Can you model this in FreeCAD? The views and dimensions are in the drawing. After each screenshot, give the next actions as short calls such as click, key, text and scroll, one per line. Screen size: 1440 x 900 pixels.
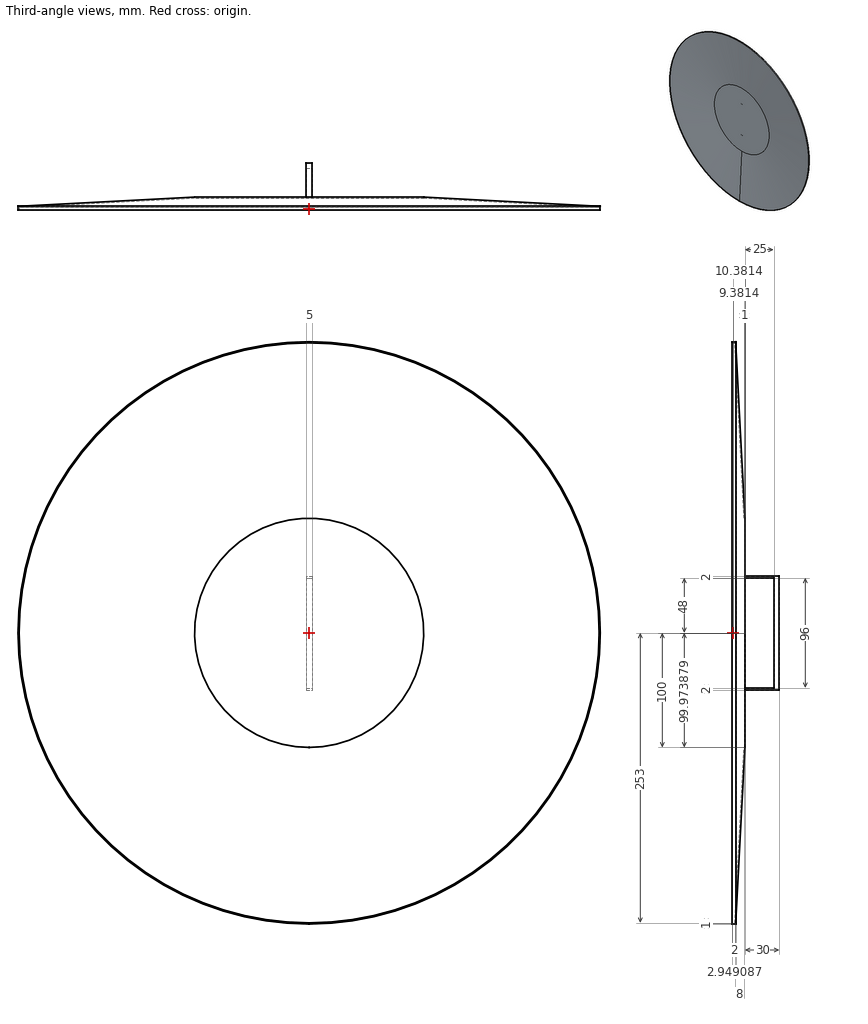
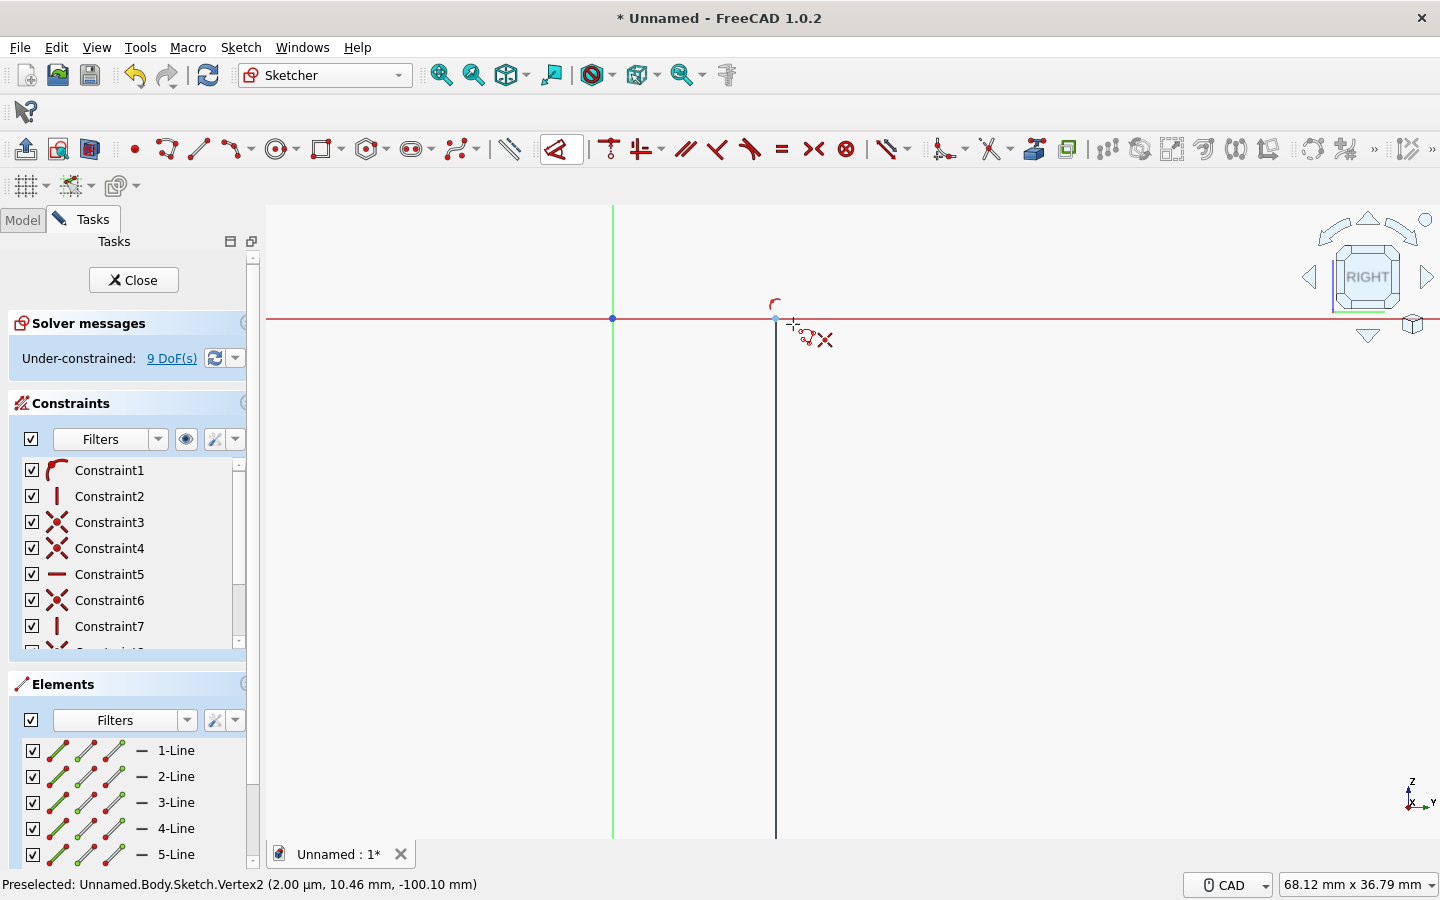
click(792, 328)
click(776, 319)
key(Escape)
key(Escape)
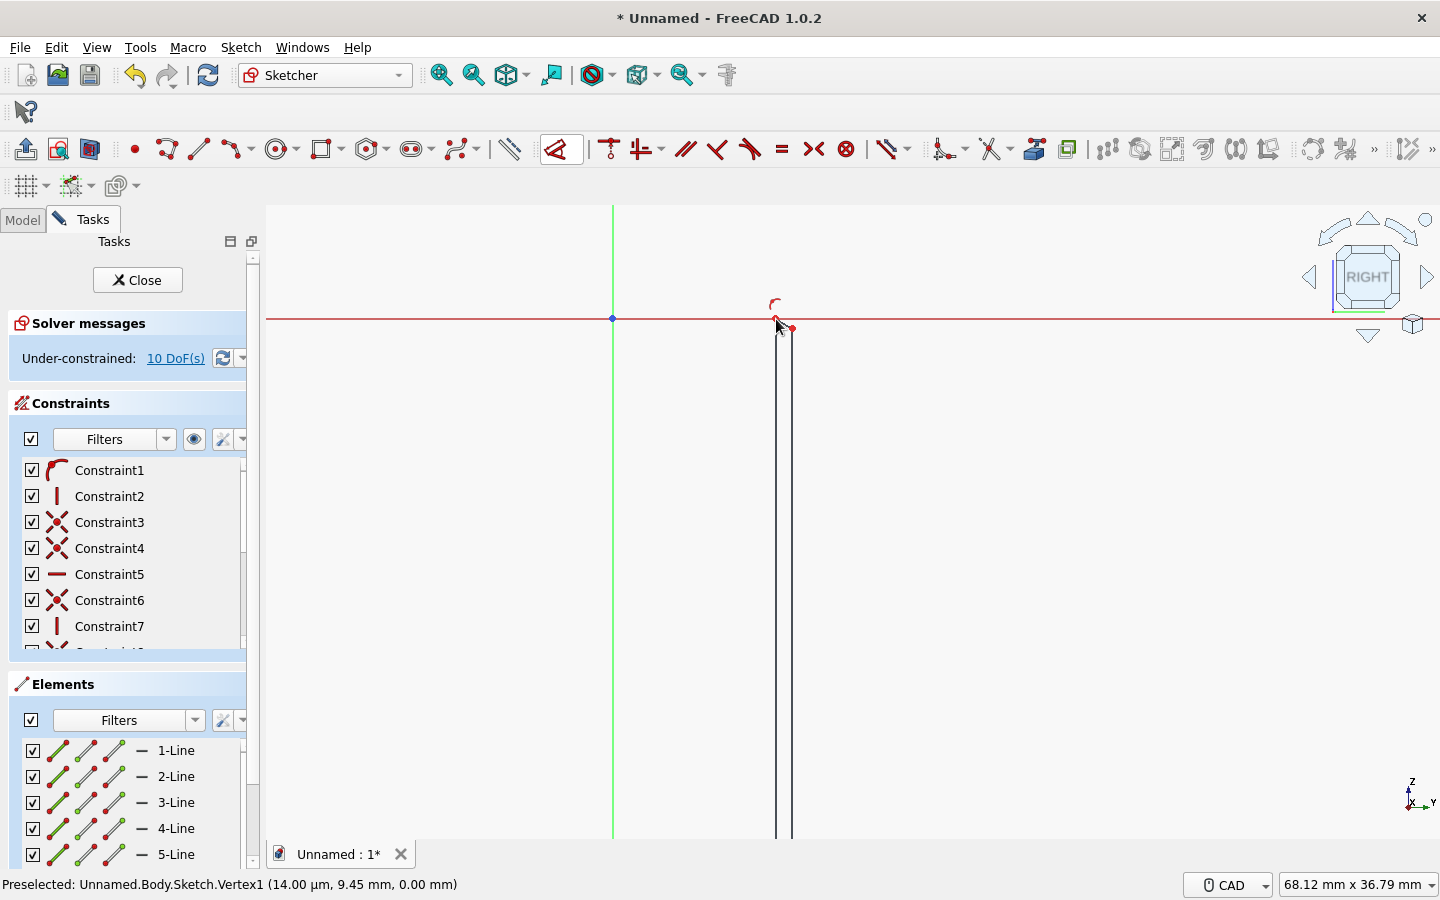
scroll(782, 323, up, 2)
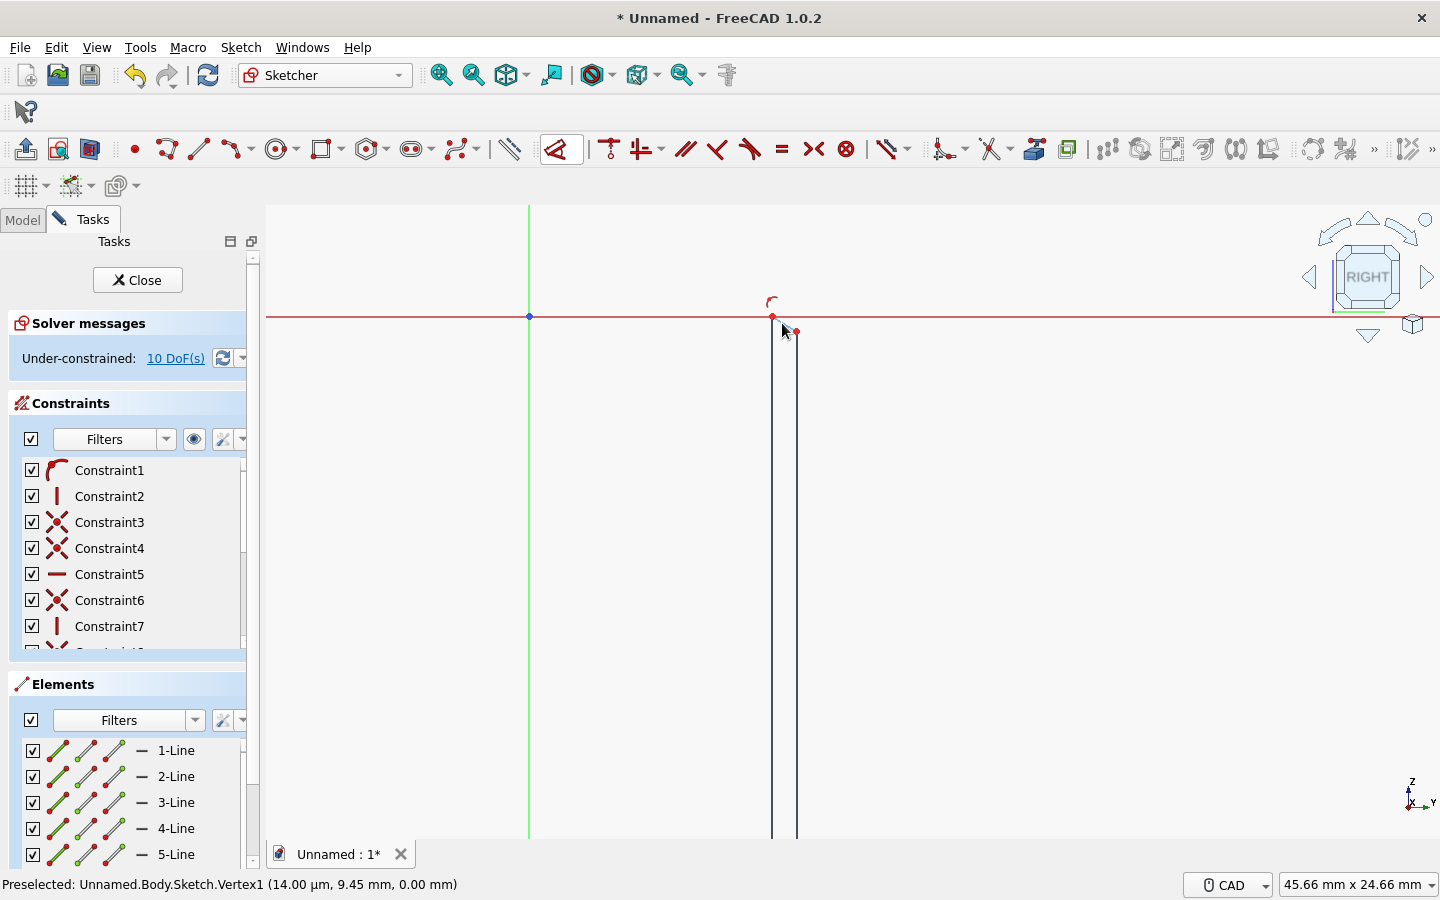
click(782, 323)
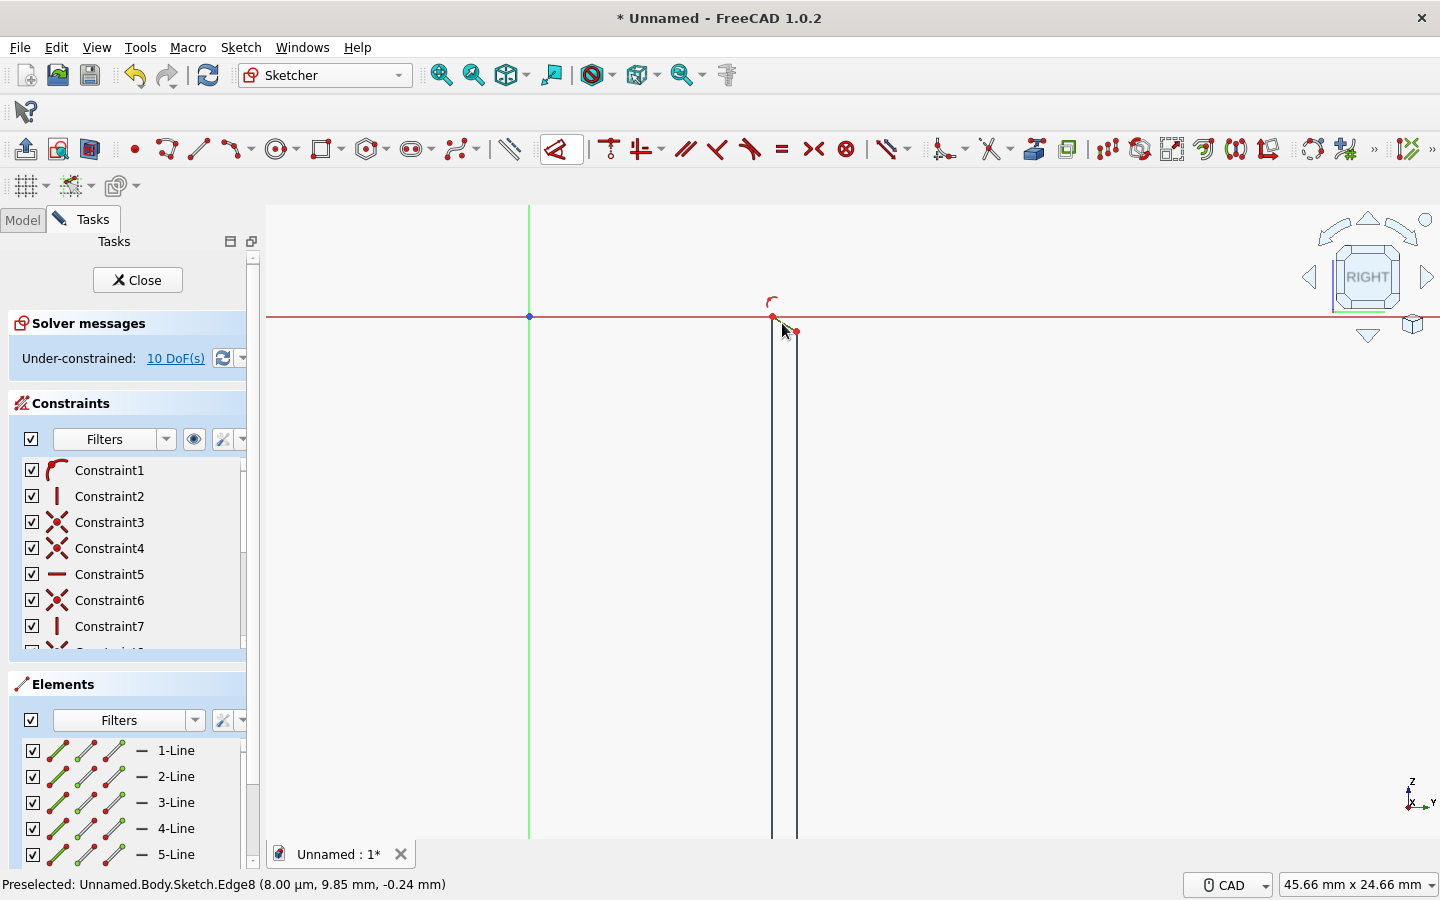
click(664, 150)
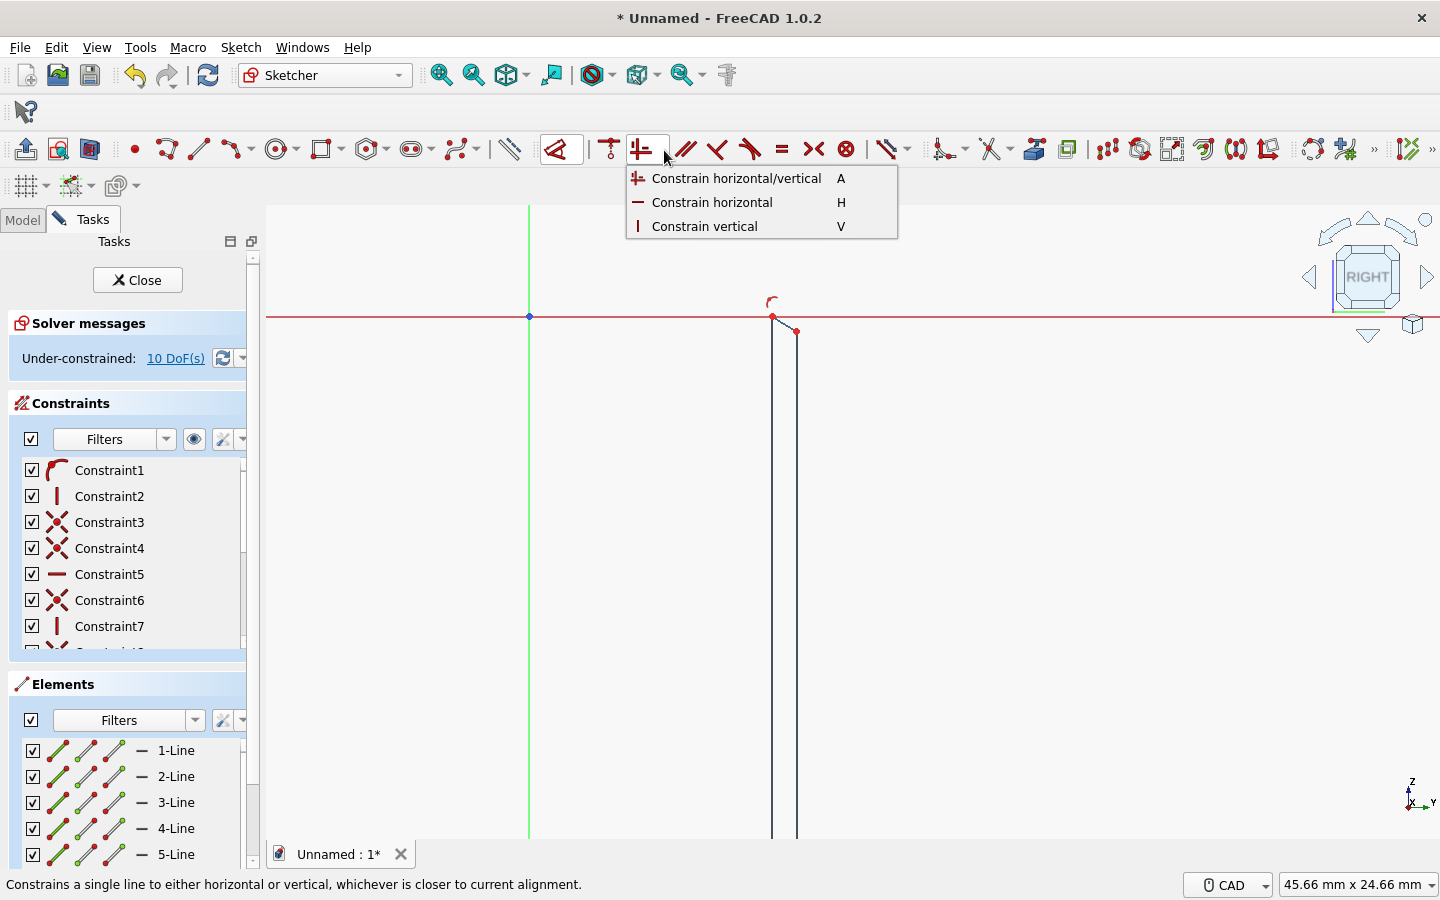
click(762, 202)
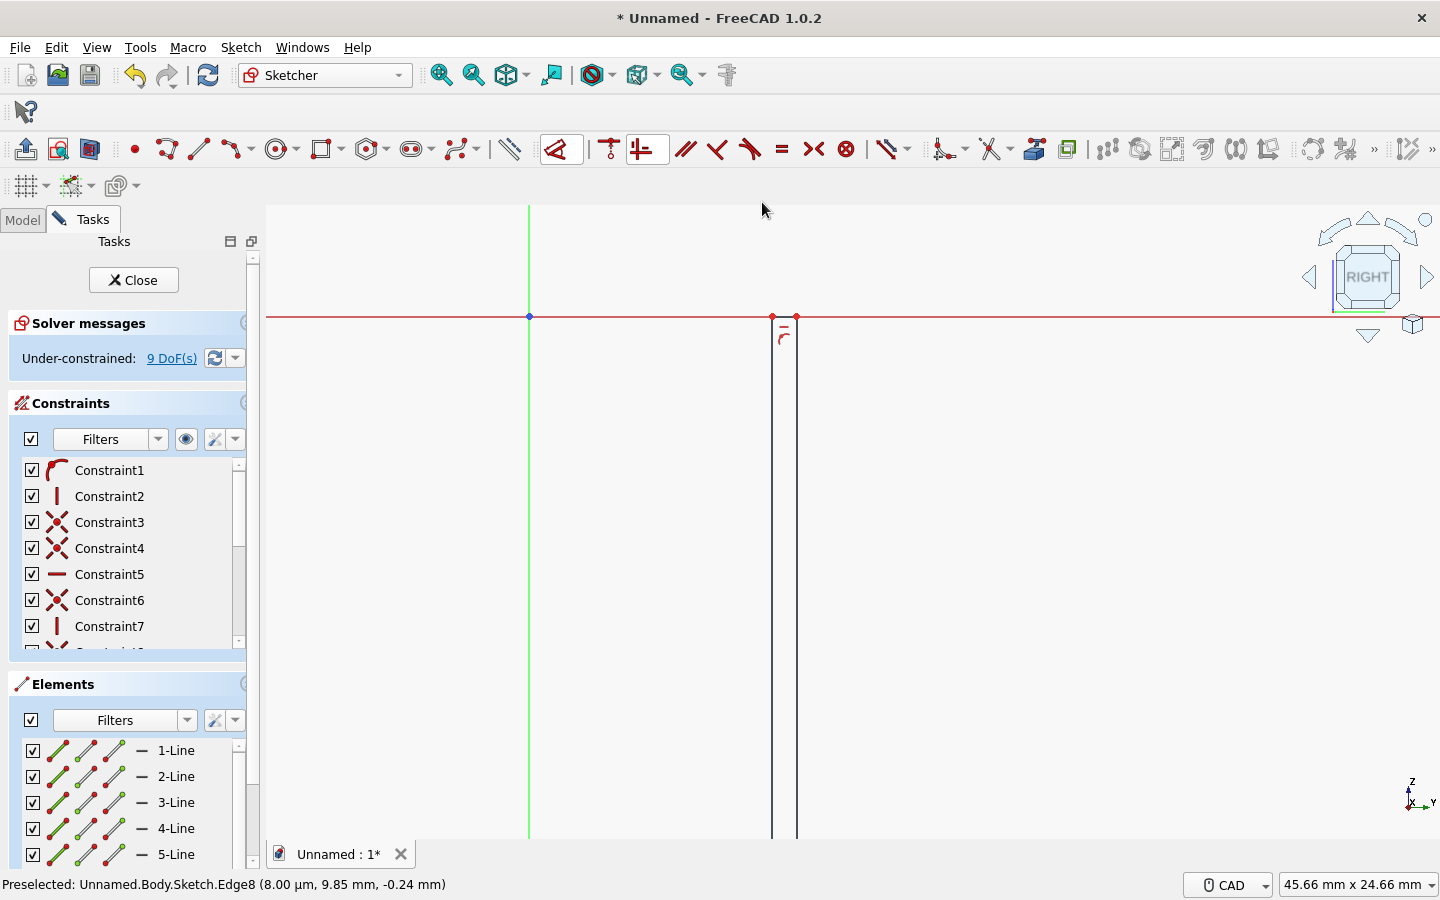
key(d)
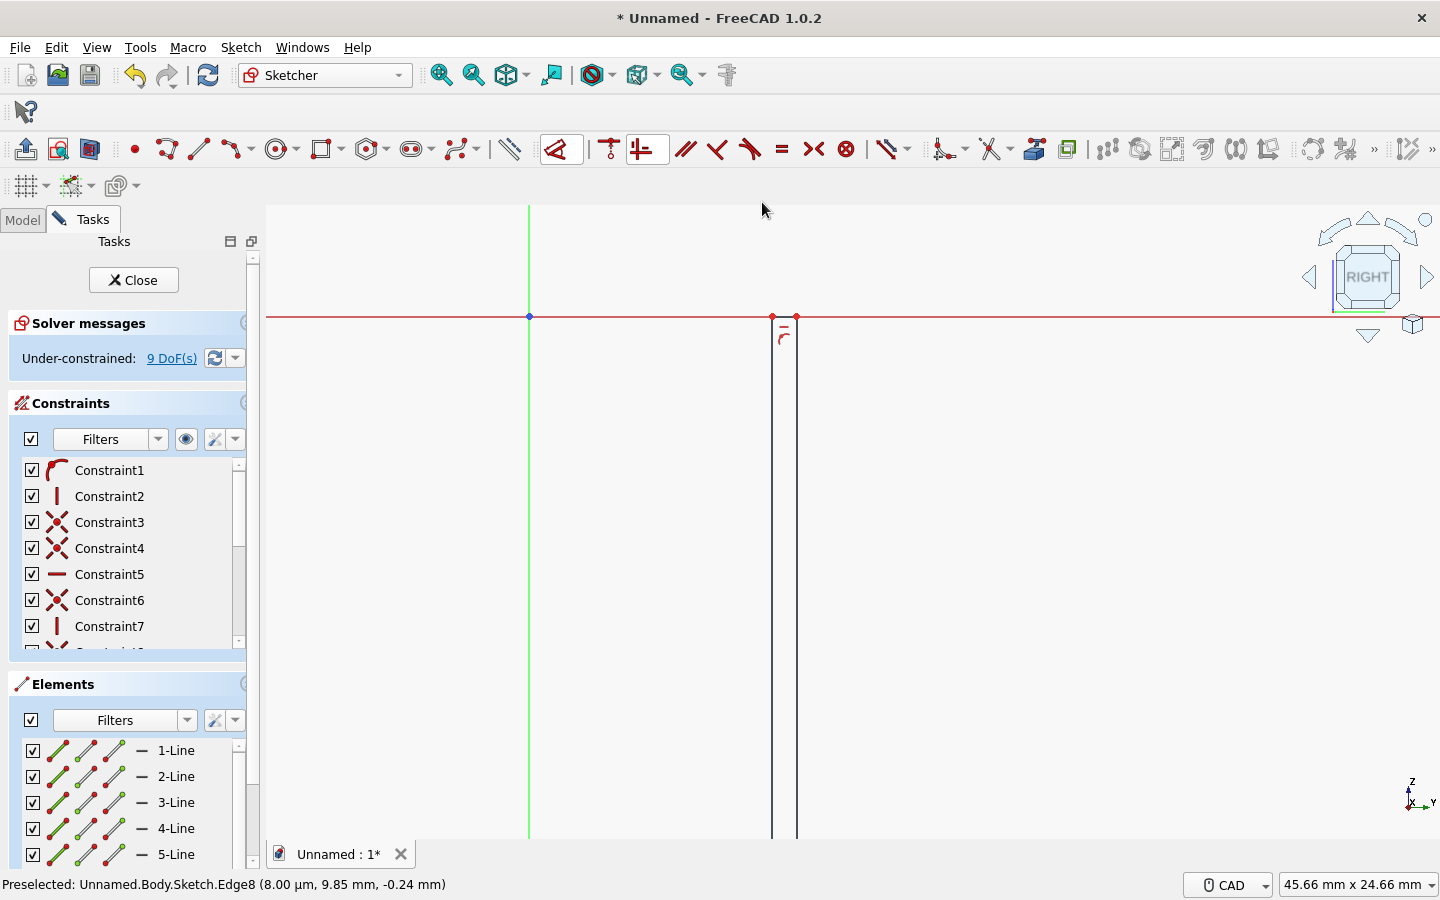
scroll(793, 324, down, 14)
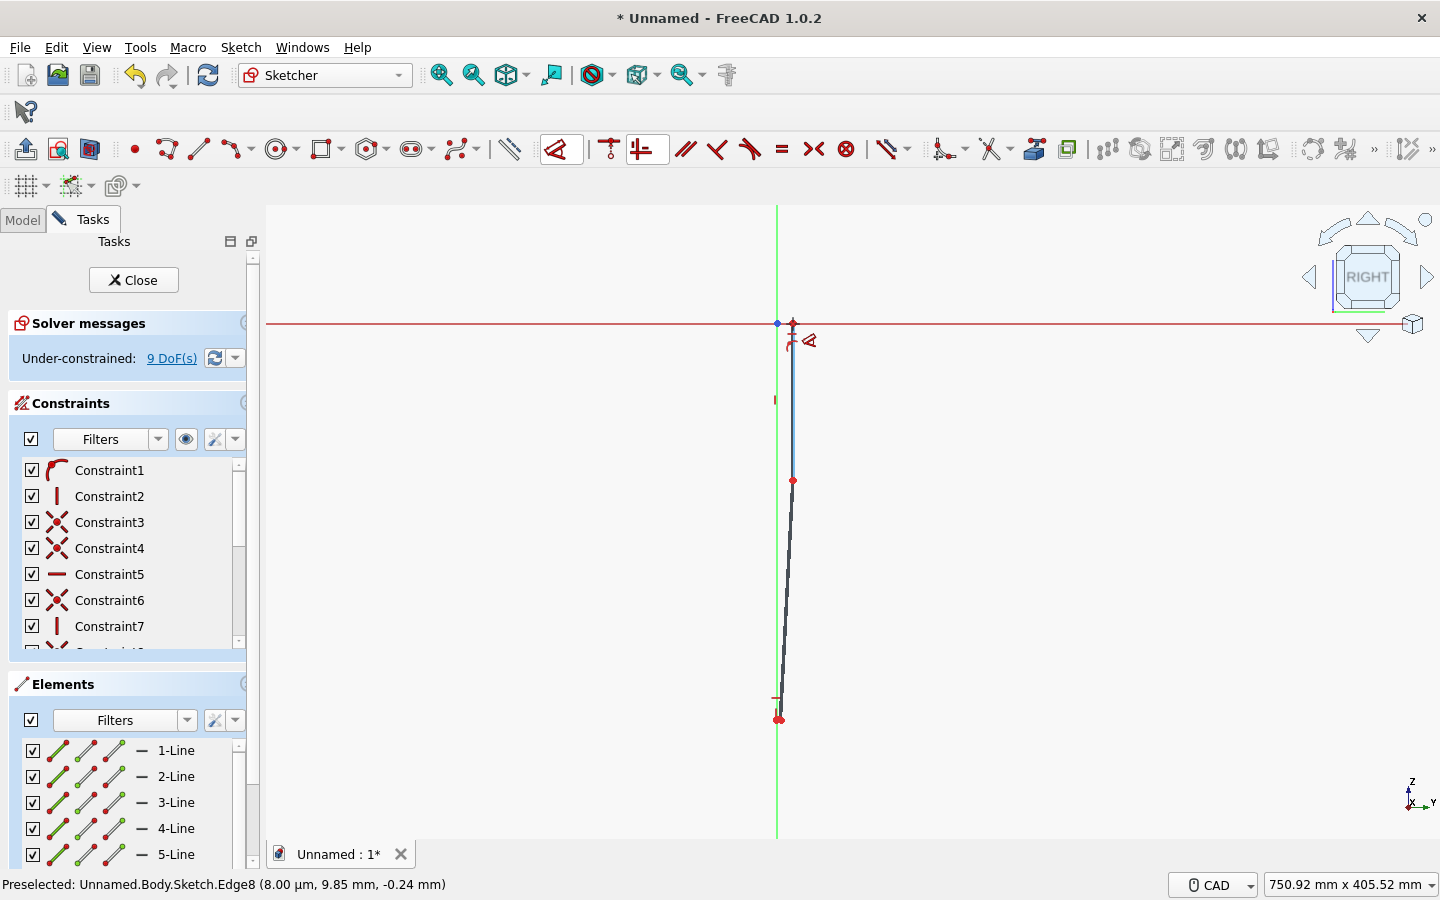
scroll(779, 719, up, 14)